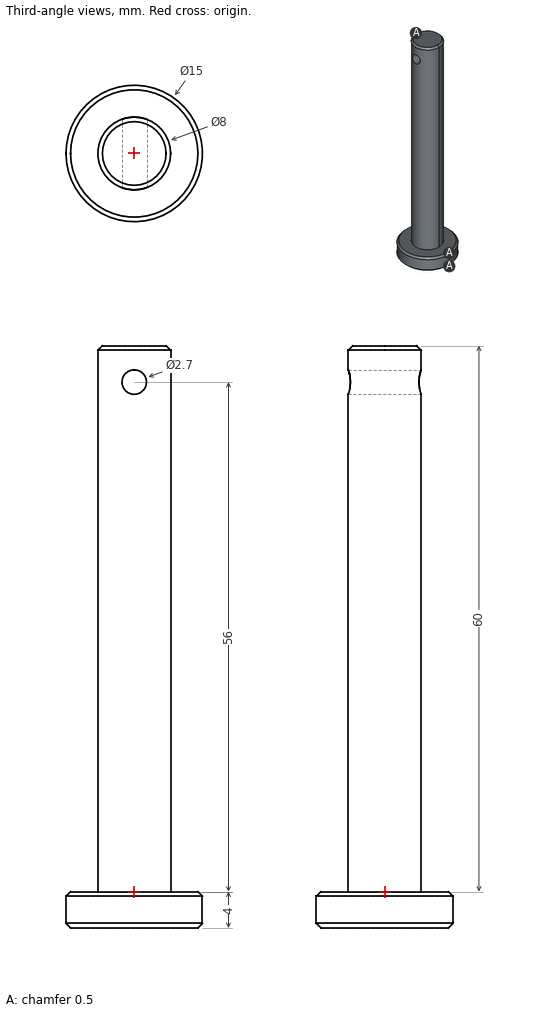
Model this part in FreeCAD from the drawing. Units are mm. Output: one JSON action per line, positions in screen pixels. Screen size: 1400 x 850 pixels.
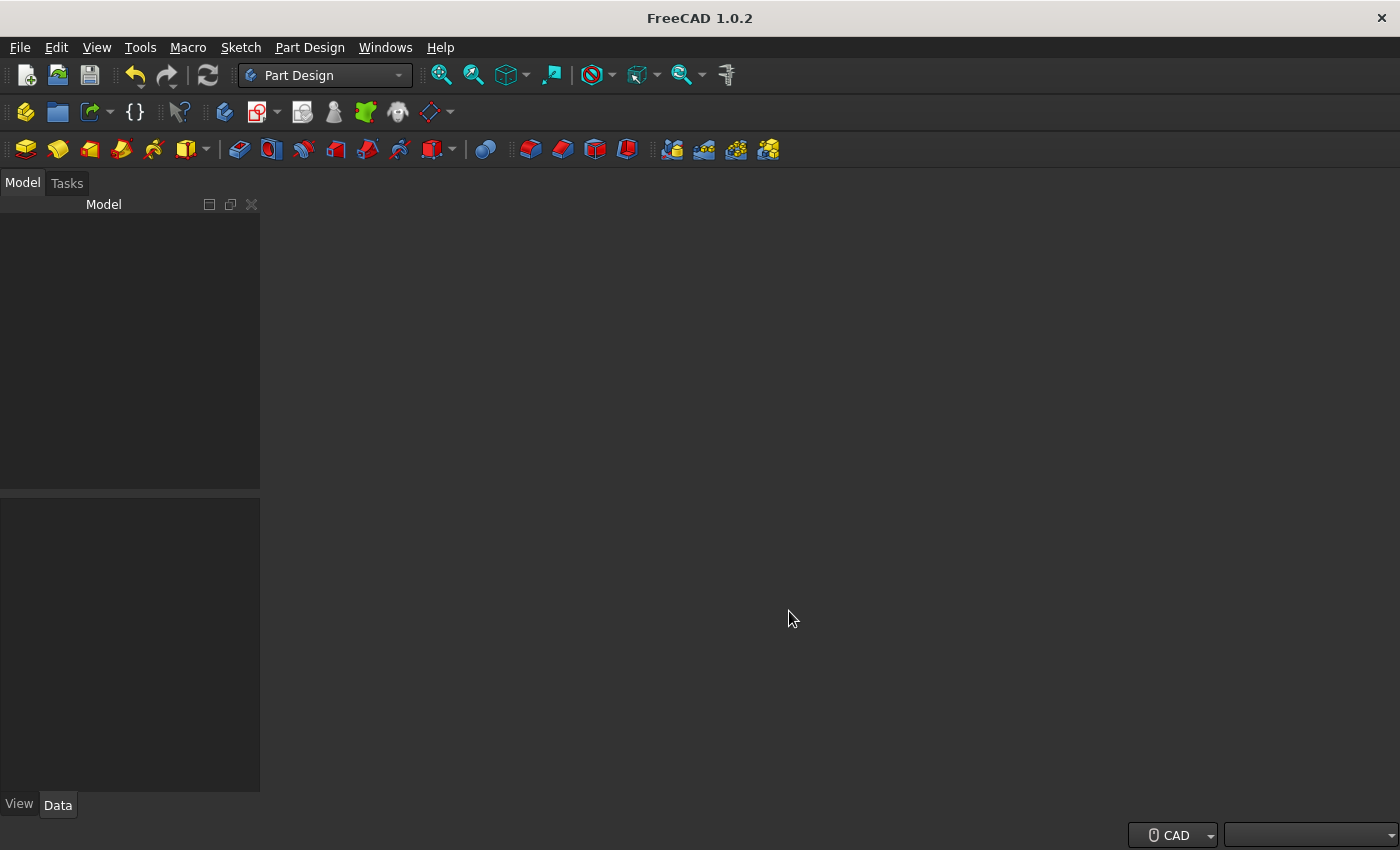
{"action": "left_click", "coordinate": [26, 76]}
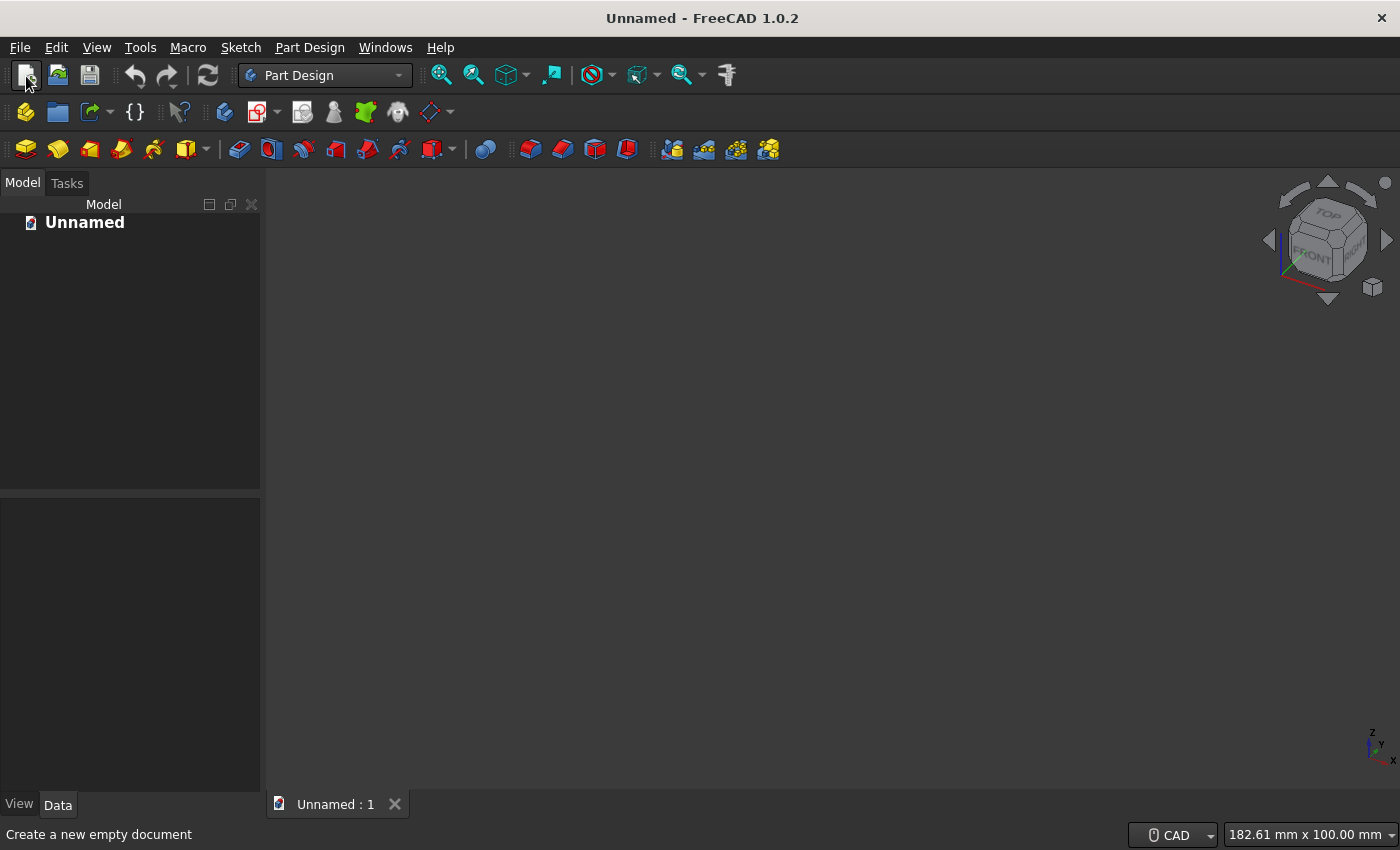
{"action": "left_click", "coordinate": [258, 112]}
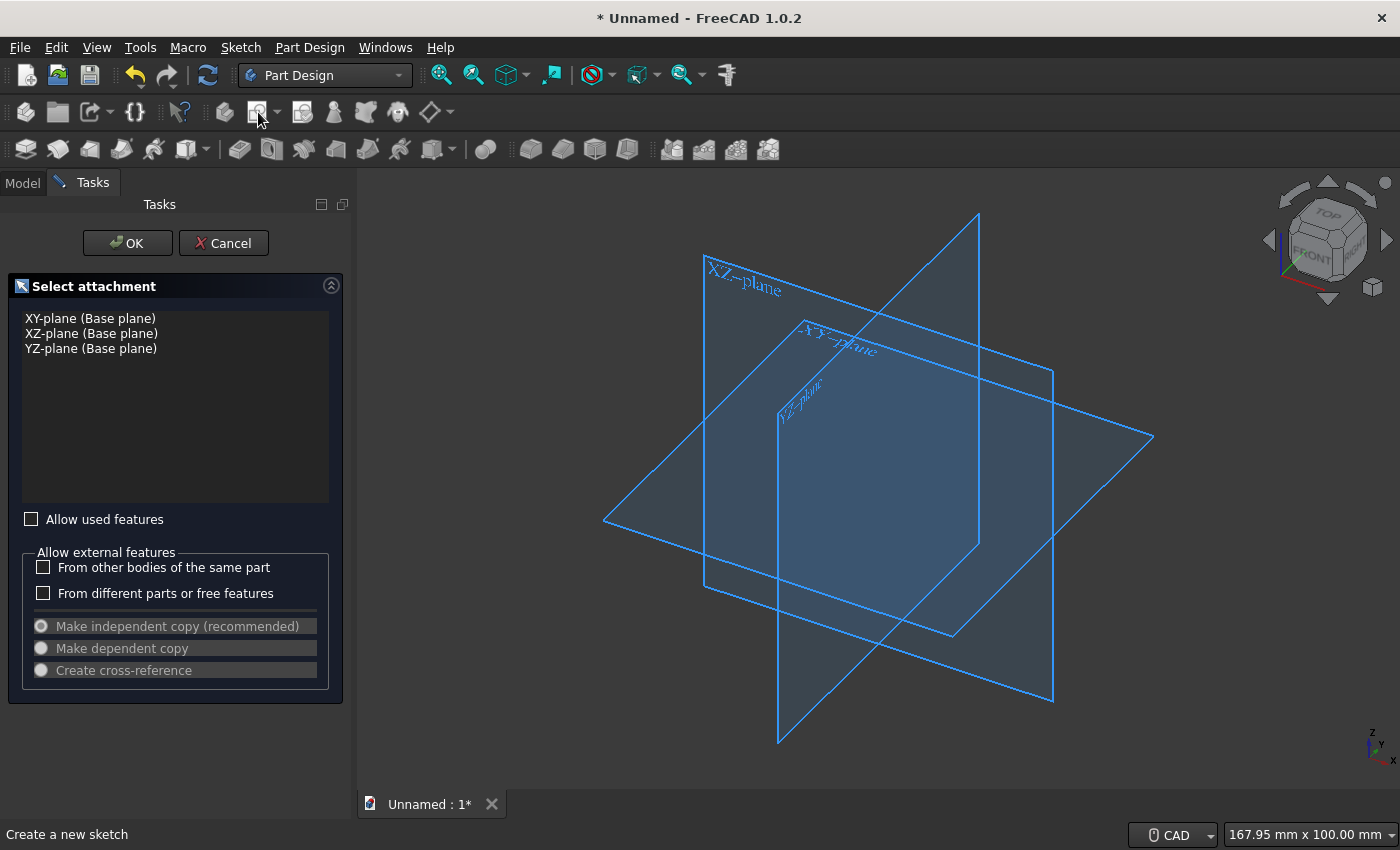
{"action": "left_click", "coordinate": [82, 318]}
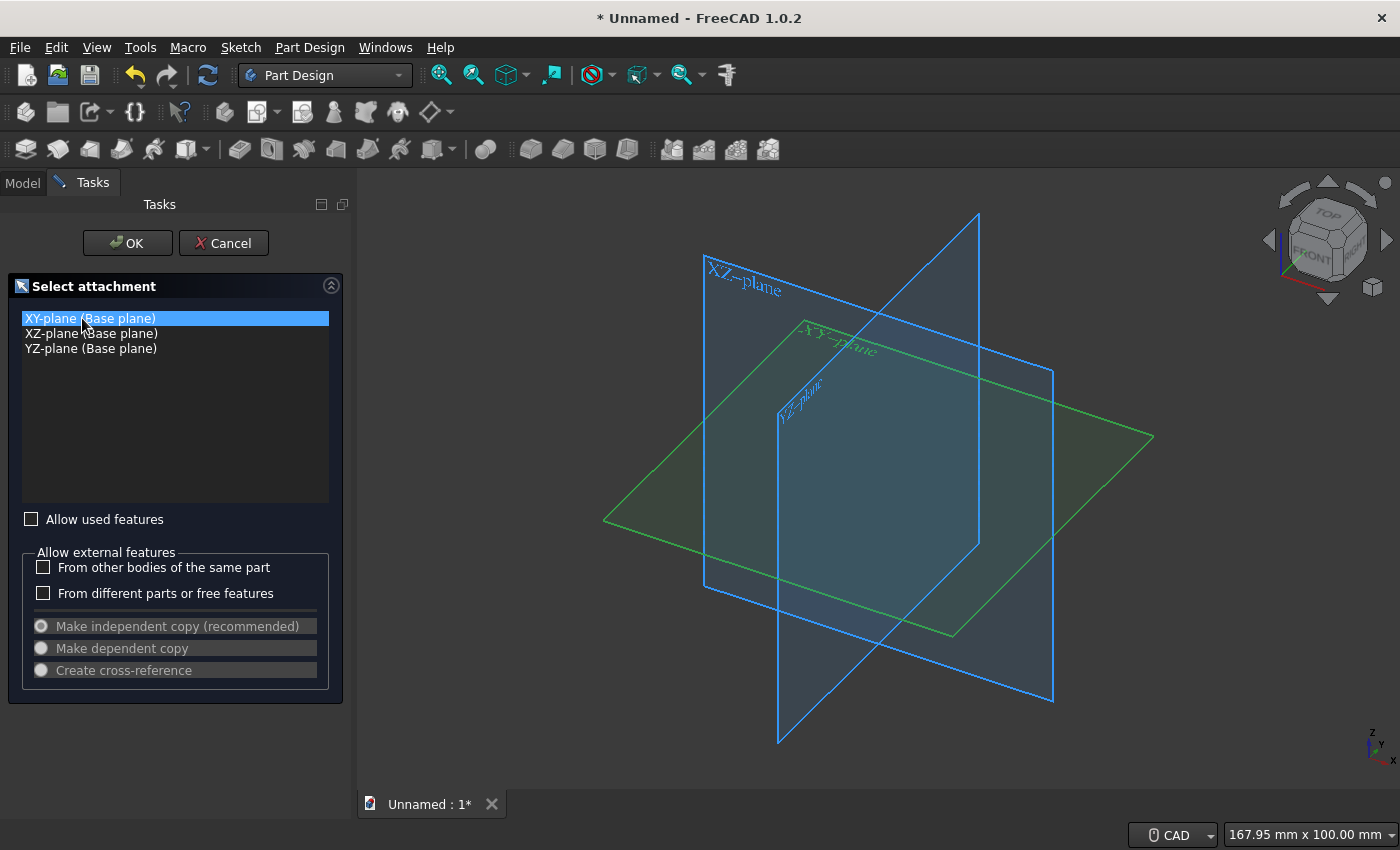
{"action": "left_click", "coordinate": [128, 243]}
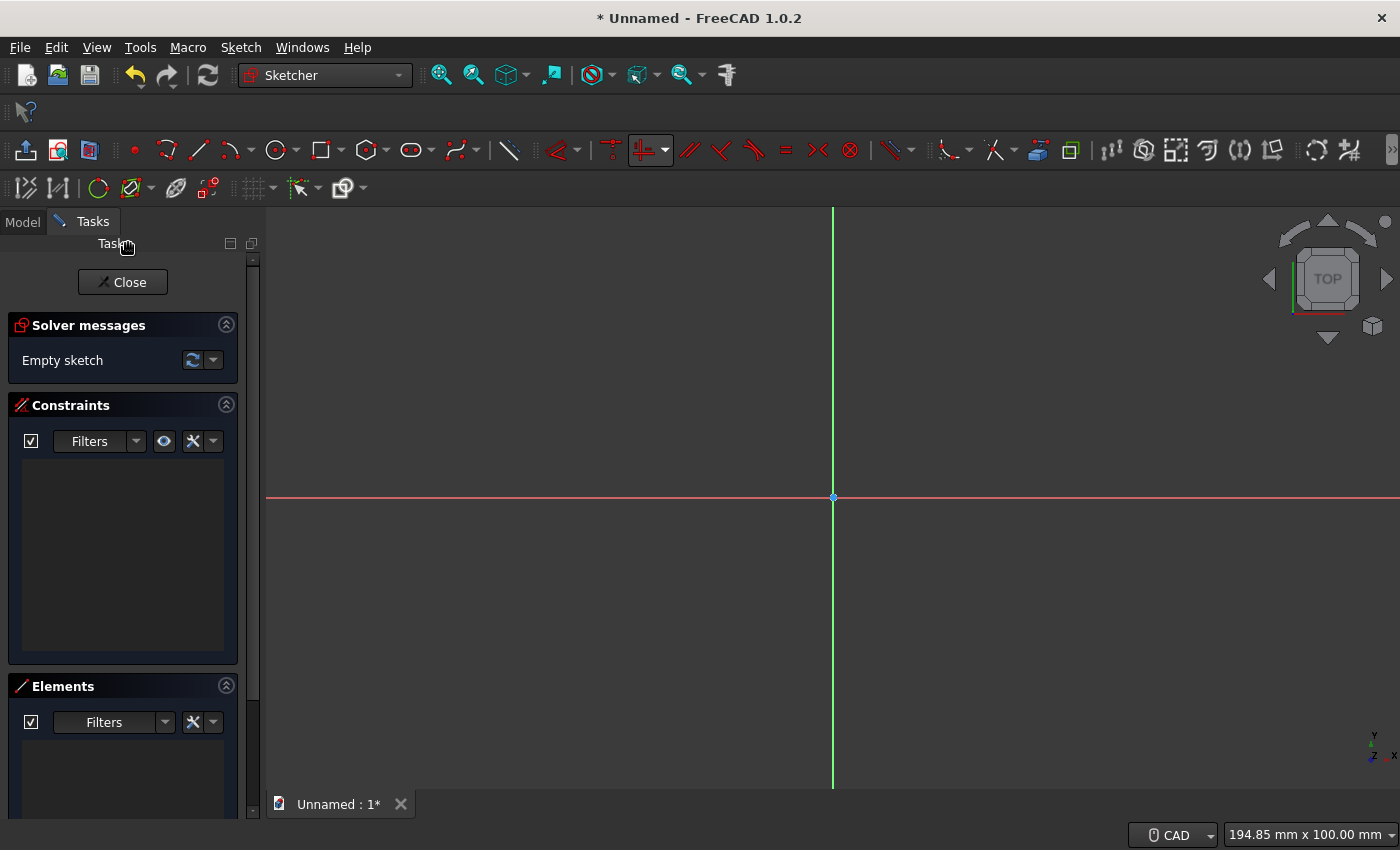
{"action": "scroll", "coordinate": [844, 498], "scroll_direction": "up", "scroll_amount": 10}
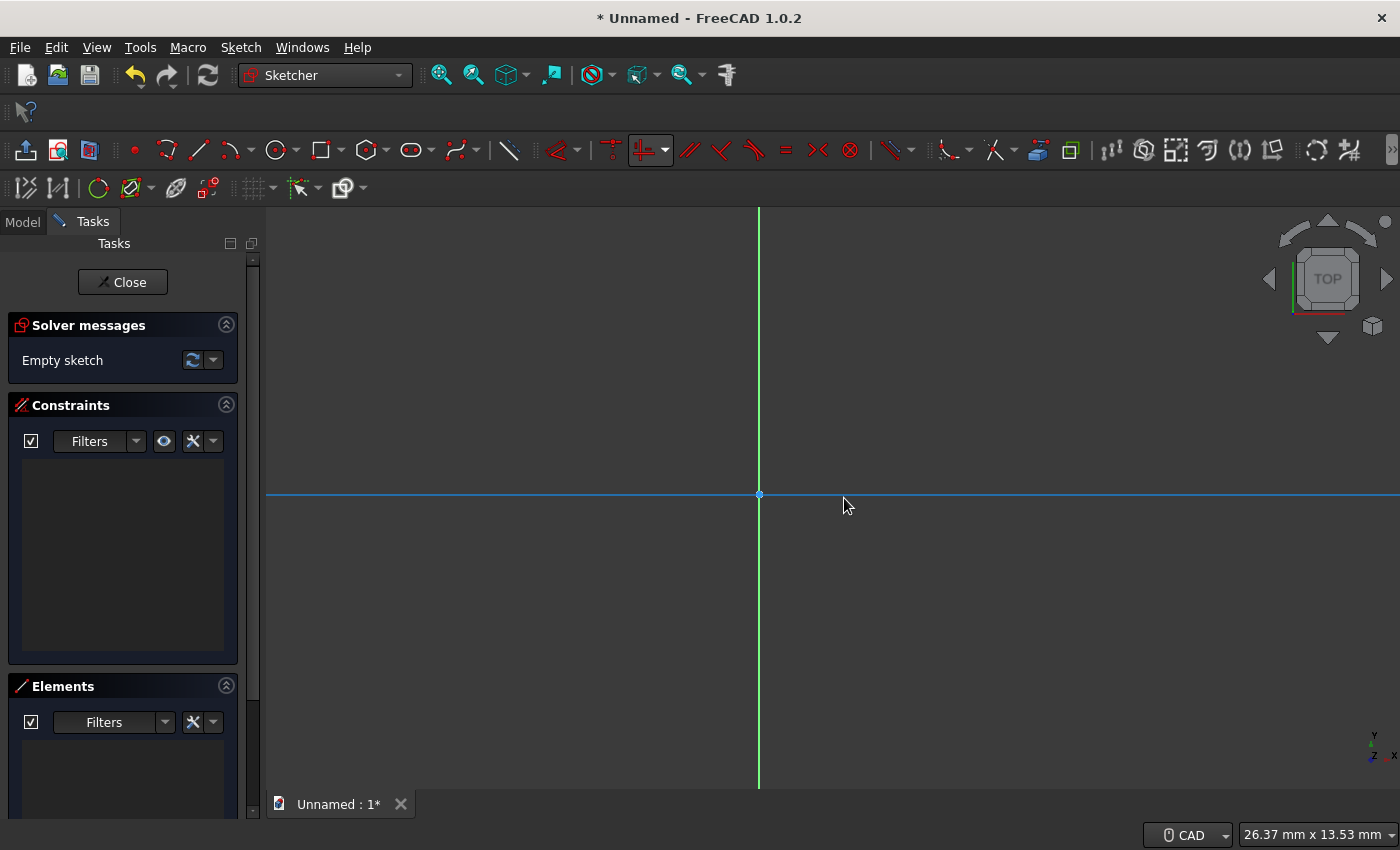
{"action": "left_click", "coordinate": [276, 150]}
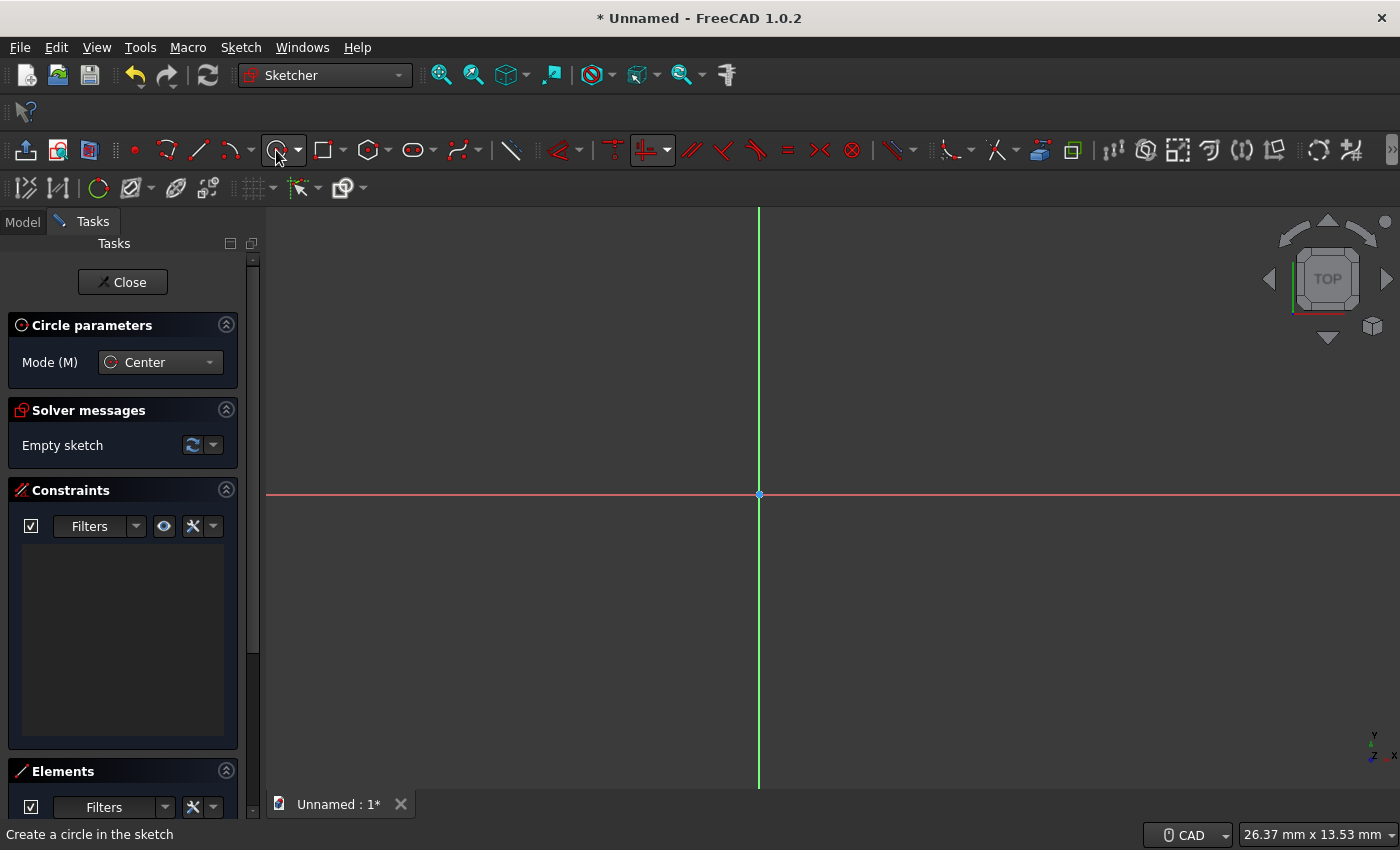
{"action": "left_click", "coordinate": [759, 495]}
{"action": "left_click", "coordinate": [881, 373]}
{"action": "key", "text": "Escape"}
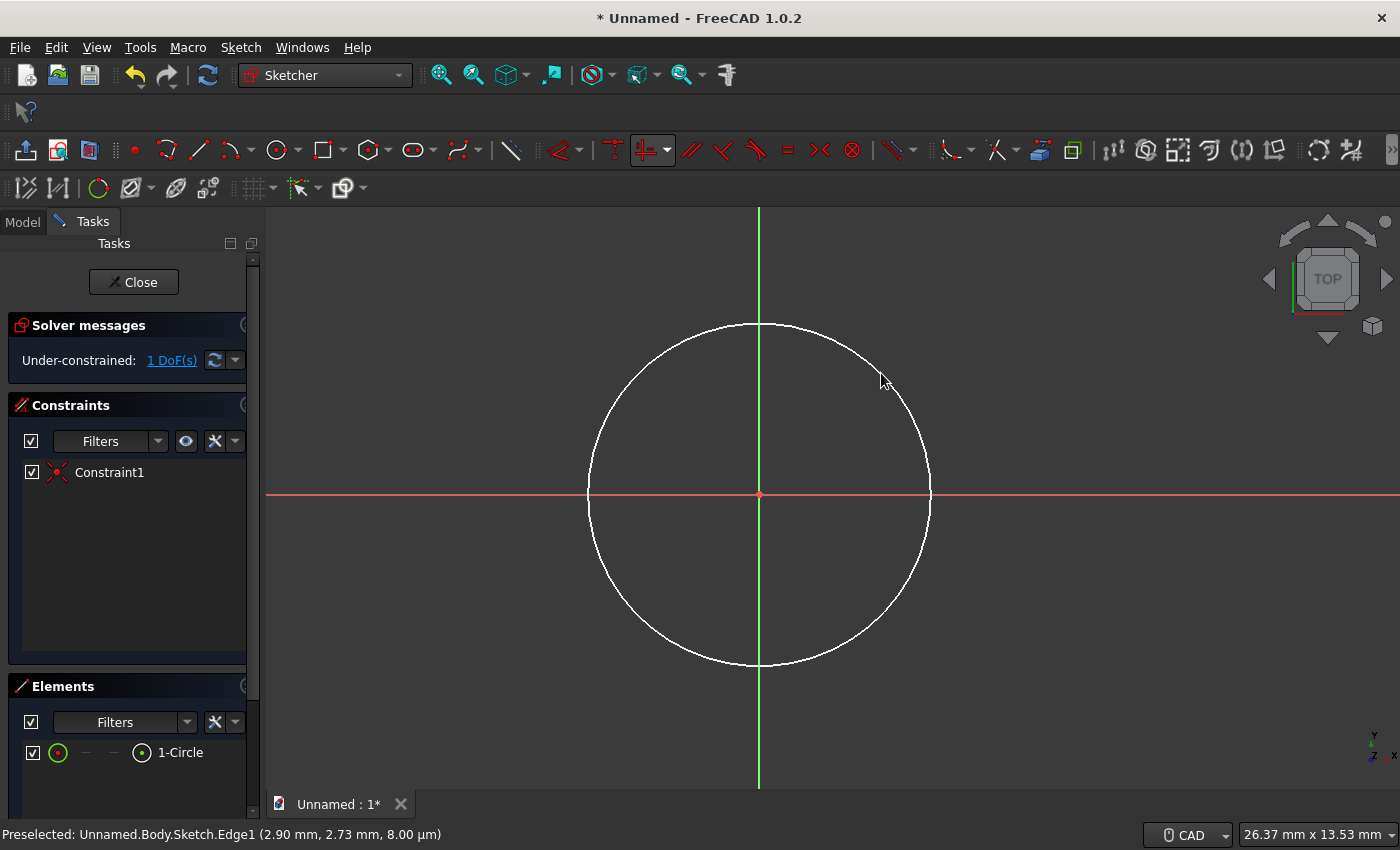
{"action": "left_click", "coordinate": [558, 150]}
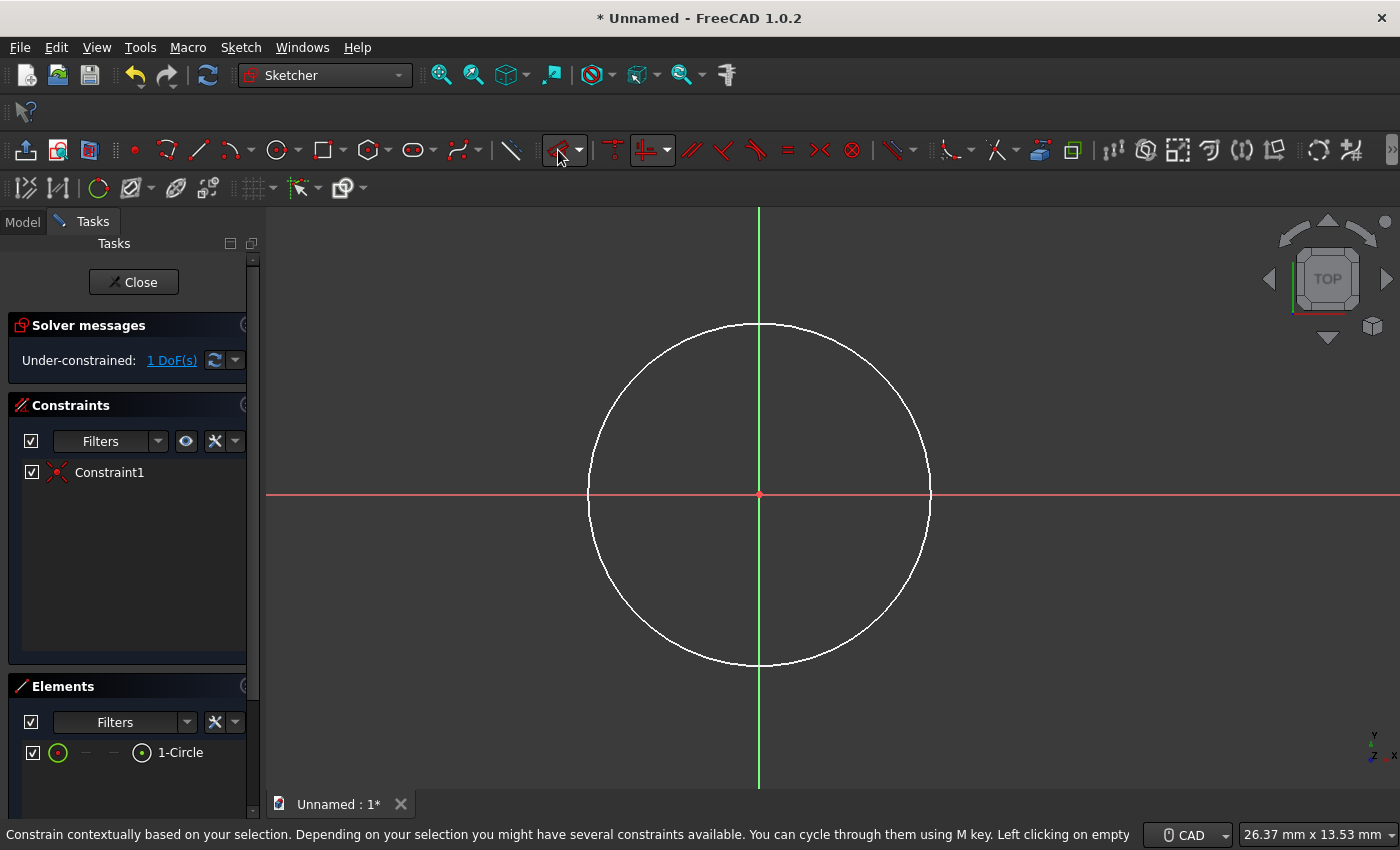
{"action": "left_click", "coordinate": [880, 373]}
{"action": "left_click", "coordinate": [903, 350]}